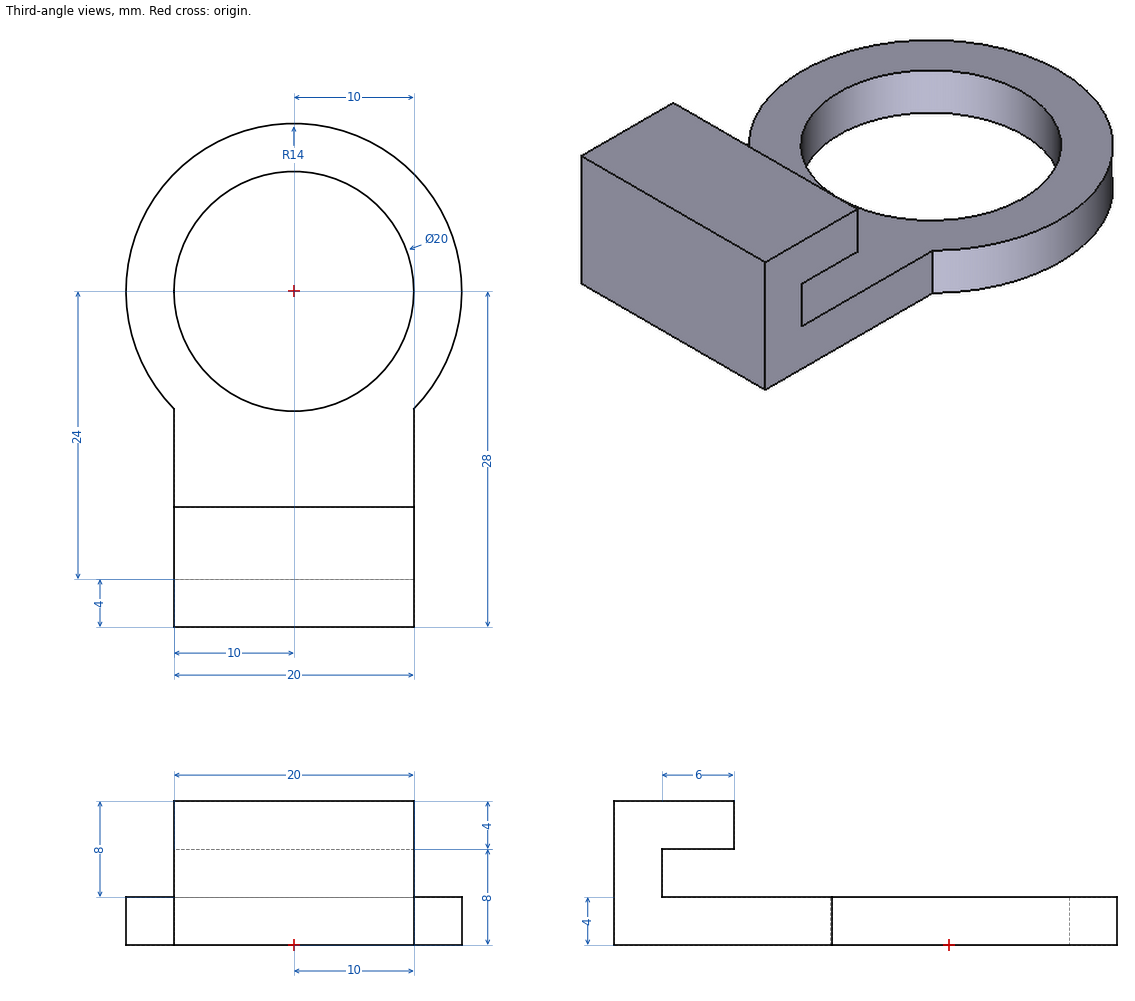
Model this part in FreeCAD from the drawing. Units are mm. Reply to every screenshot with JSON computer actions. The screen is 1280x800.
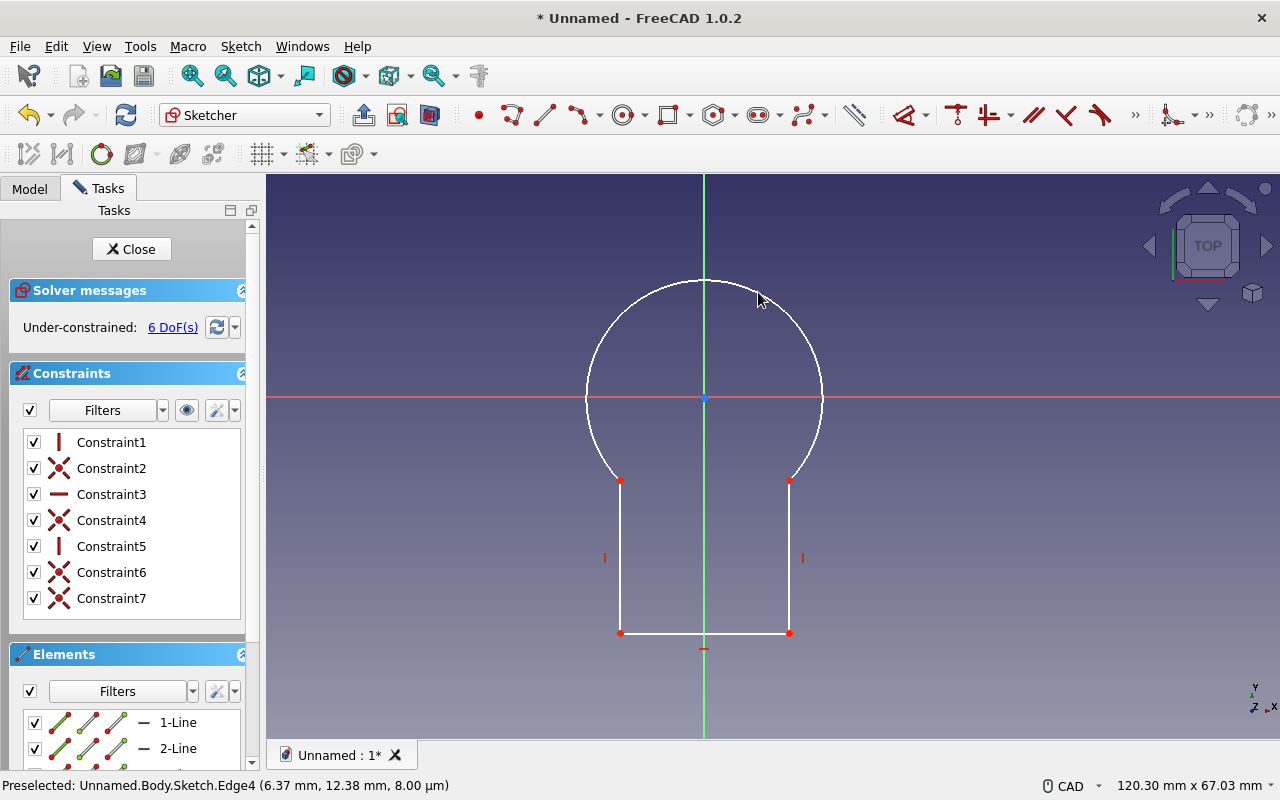
{"action": "left_click_drag", "start_coordinate": [694, 387], "coordinate": [714, 408]}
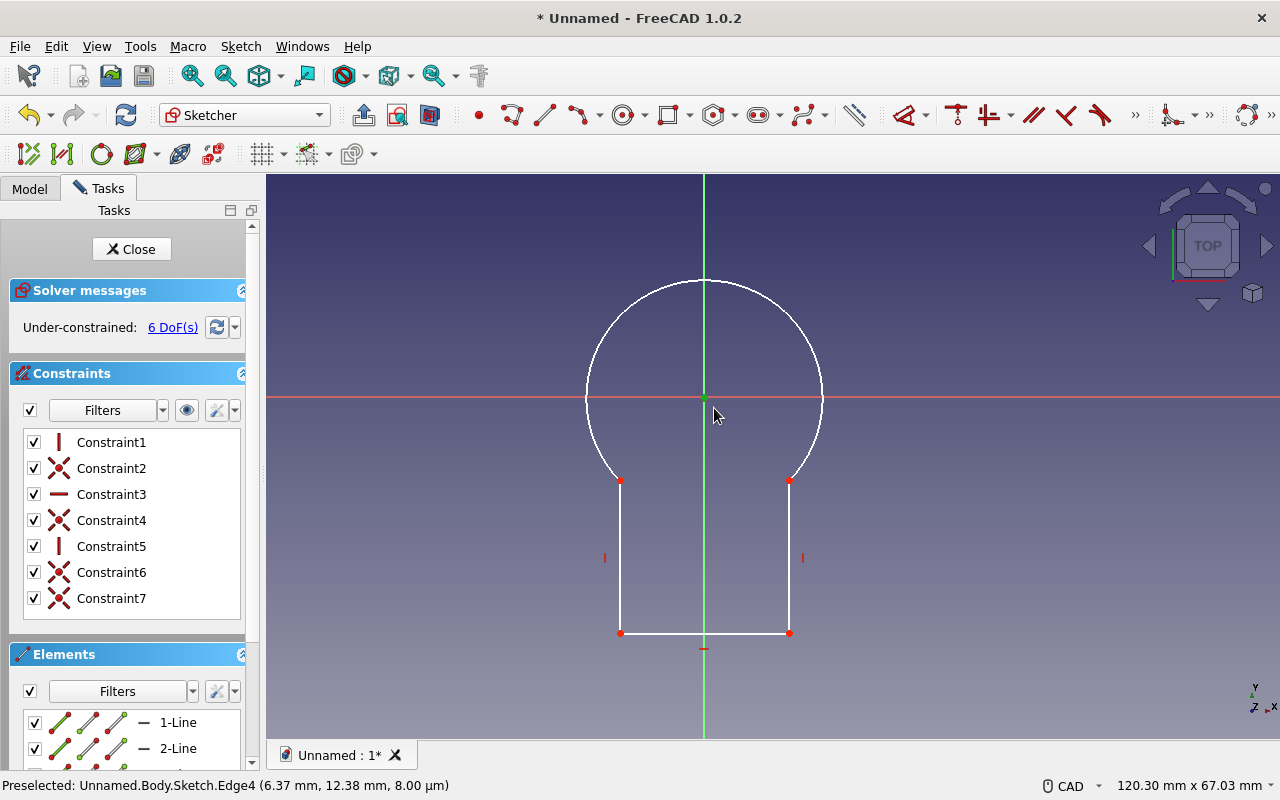
{"action": "left_click", "coordinate": [956, 116]}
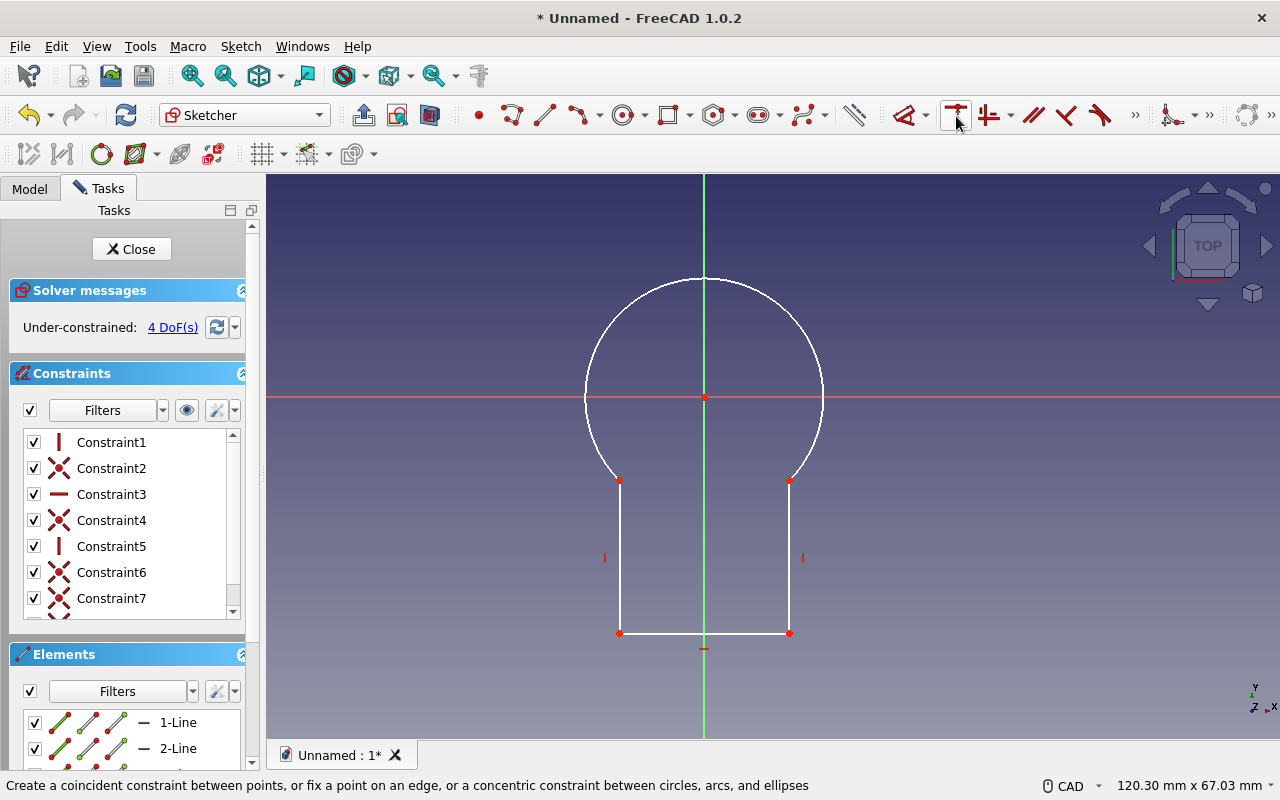
{"action": "left_click", "coordinate": [904, 116]}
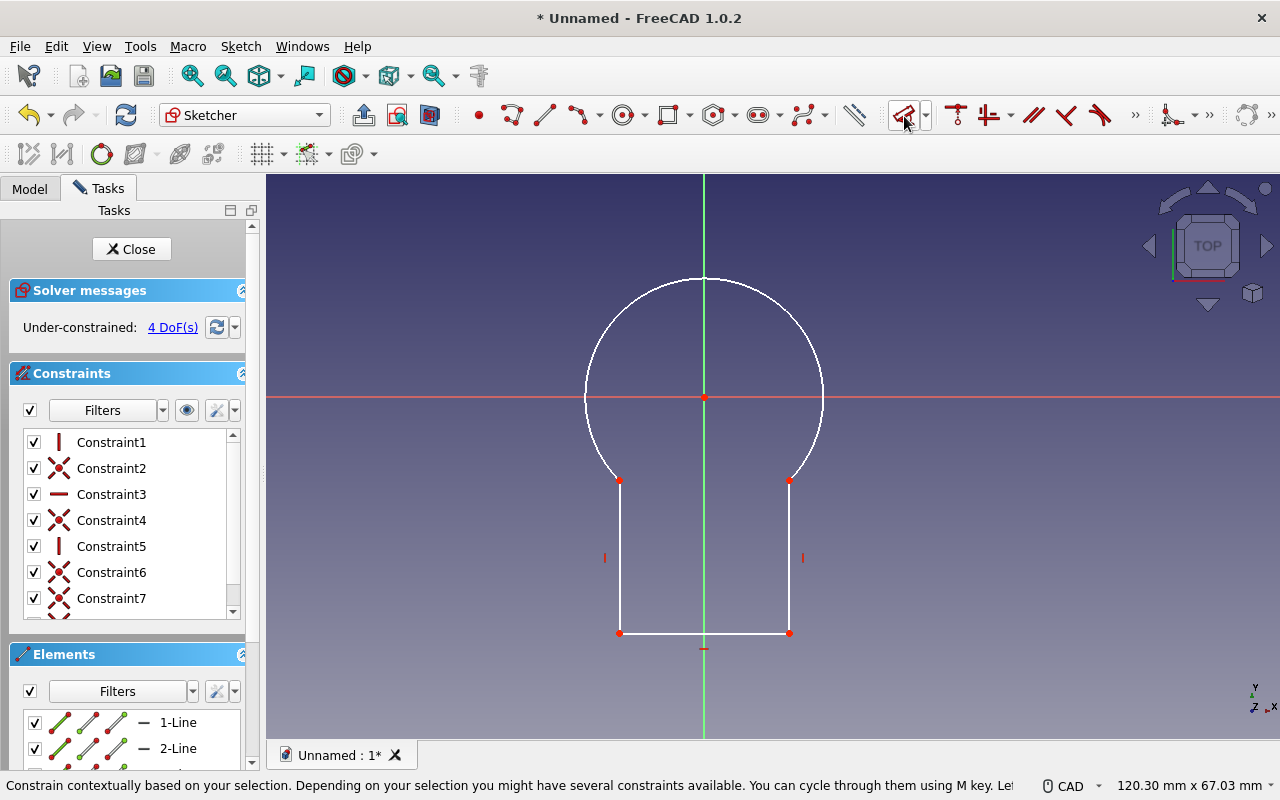
{"action": "left_click", "coordinate": [800, 327]}
{"action": "left_click", "coordinate": [826, 308]}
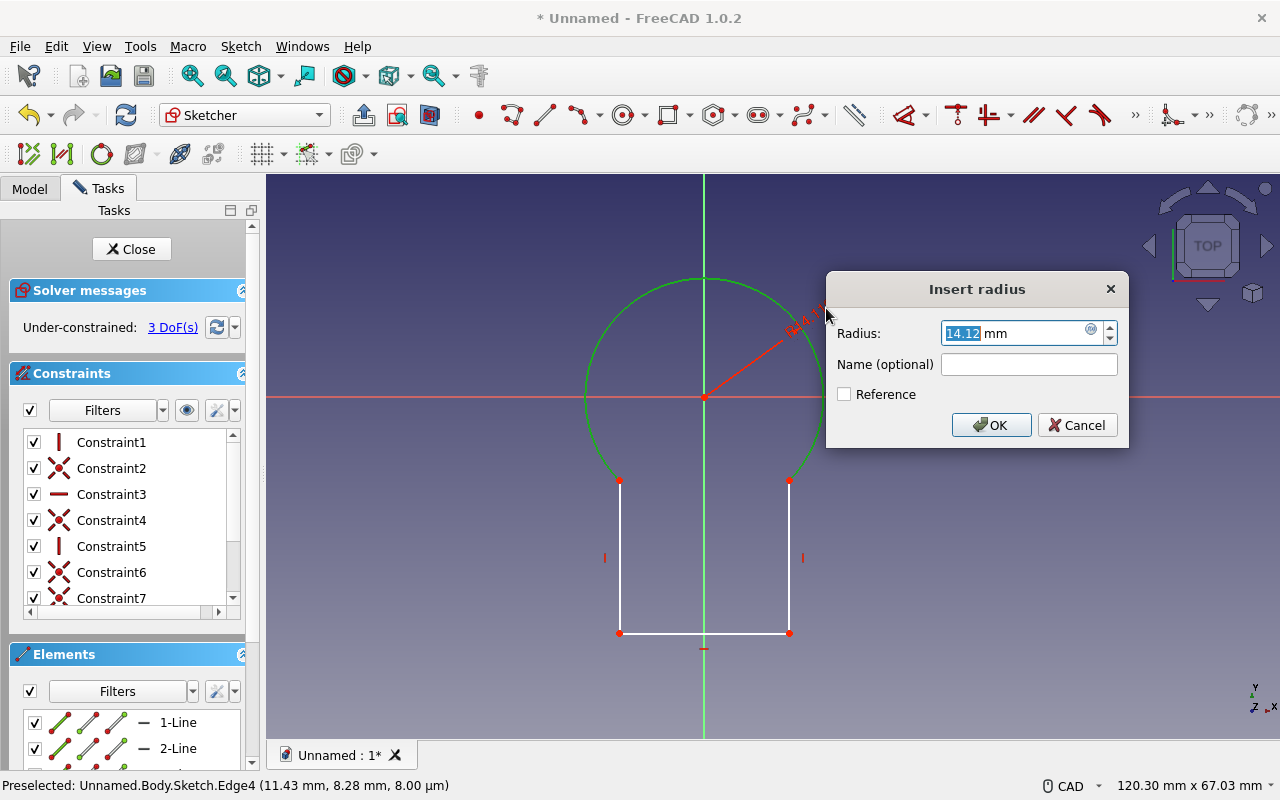
{"action": "type", "text": "14"}
{"action": "key", "text": "Return"}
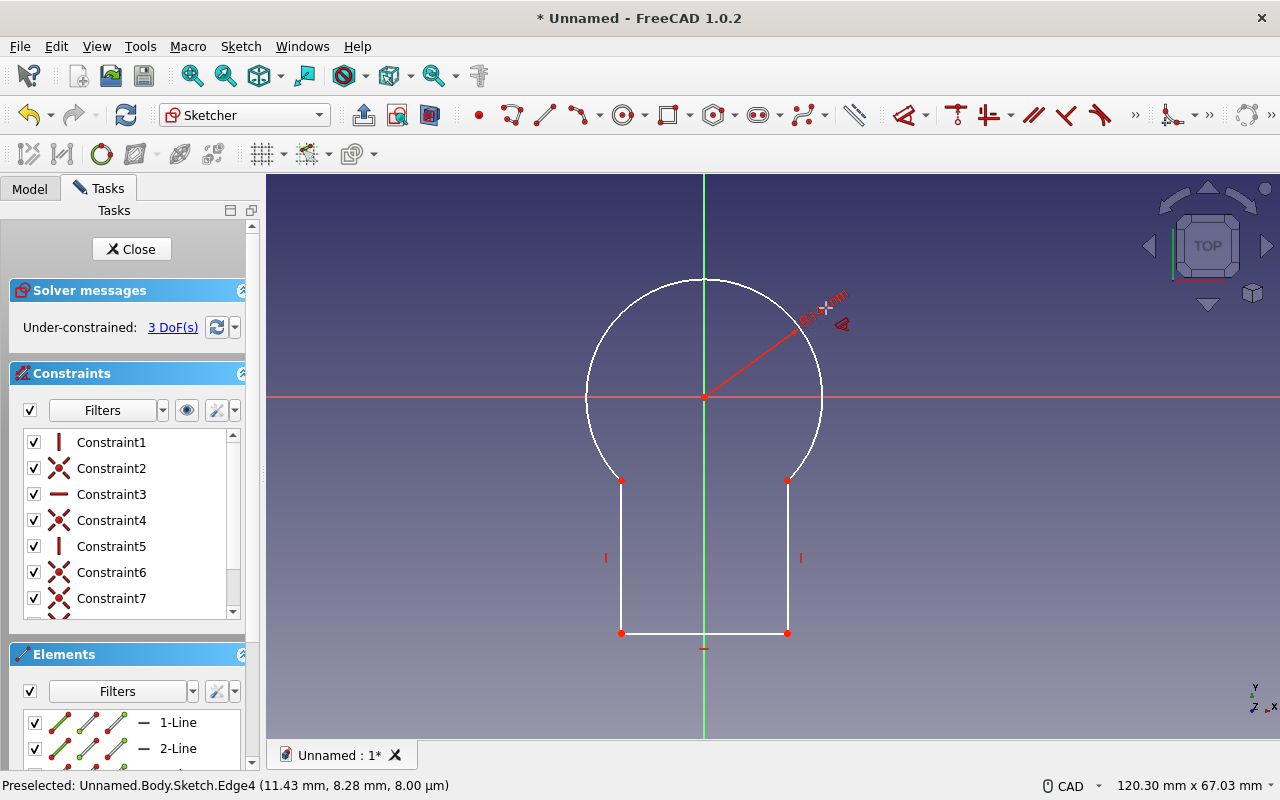
{"action": "left_click", "coordinate": [738, 634]}
{"action": "left_click", "coordinate": [666, 668]}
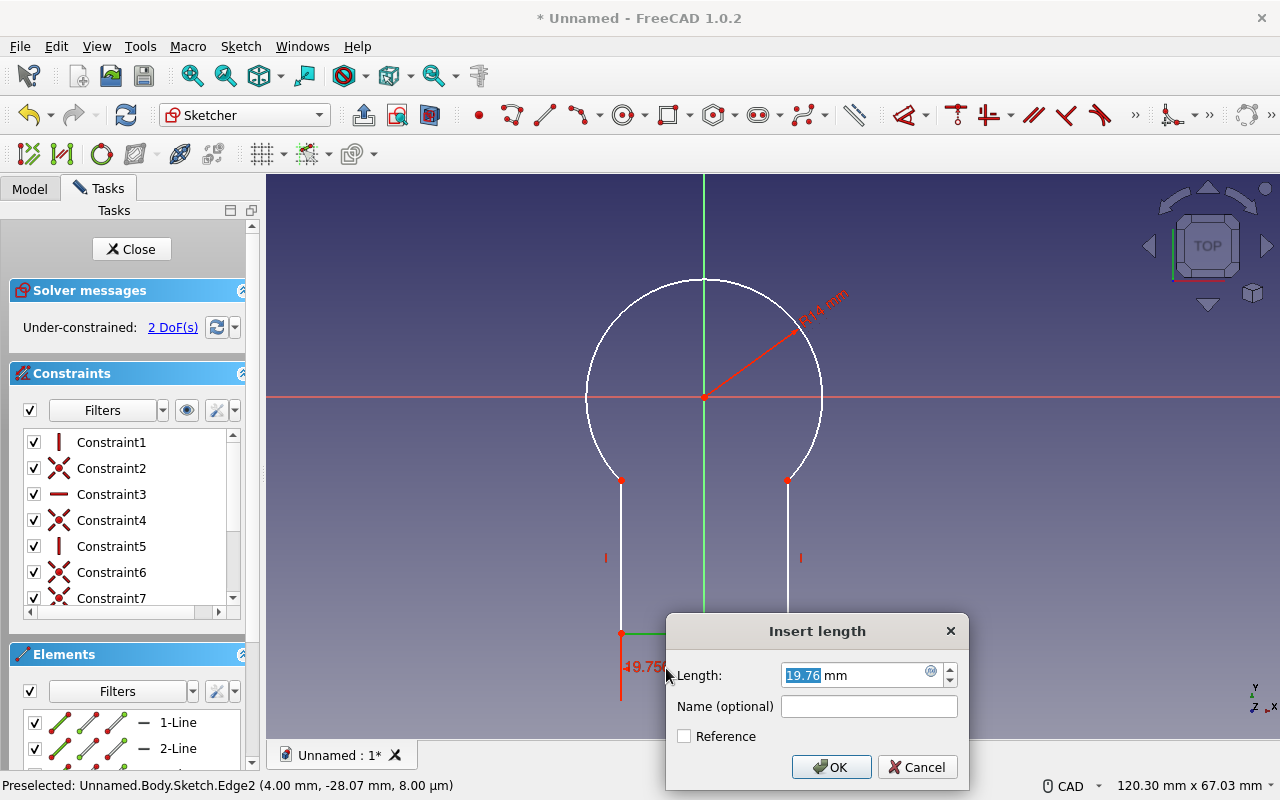
{"action": "type", "text": "20"}
{"action": "key", "text": "Return"}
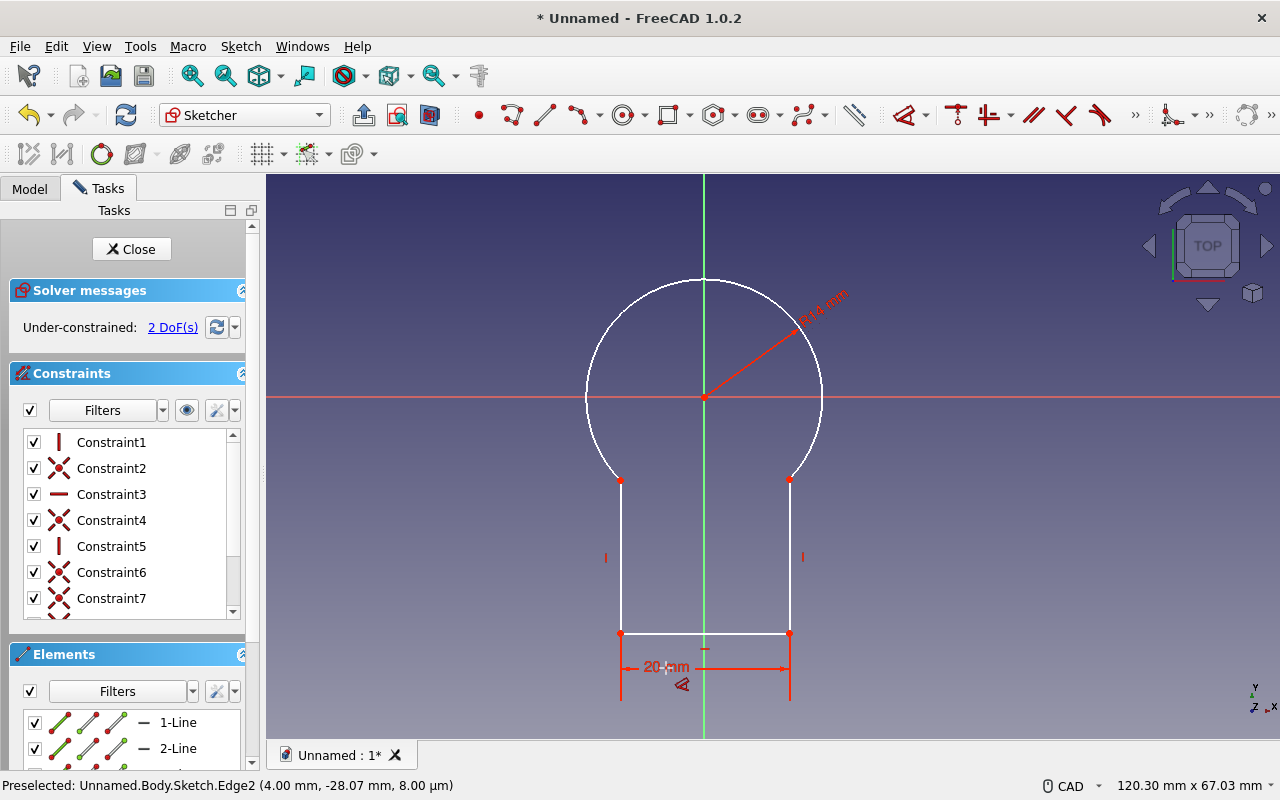
{"action": "left_click", "coordinate": [790, 479]}
{"action": "left_click", "coordinate": [747, 363]}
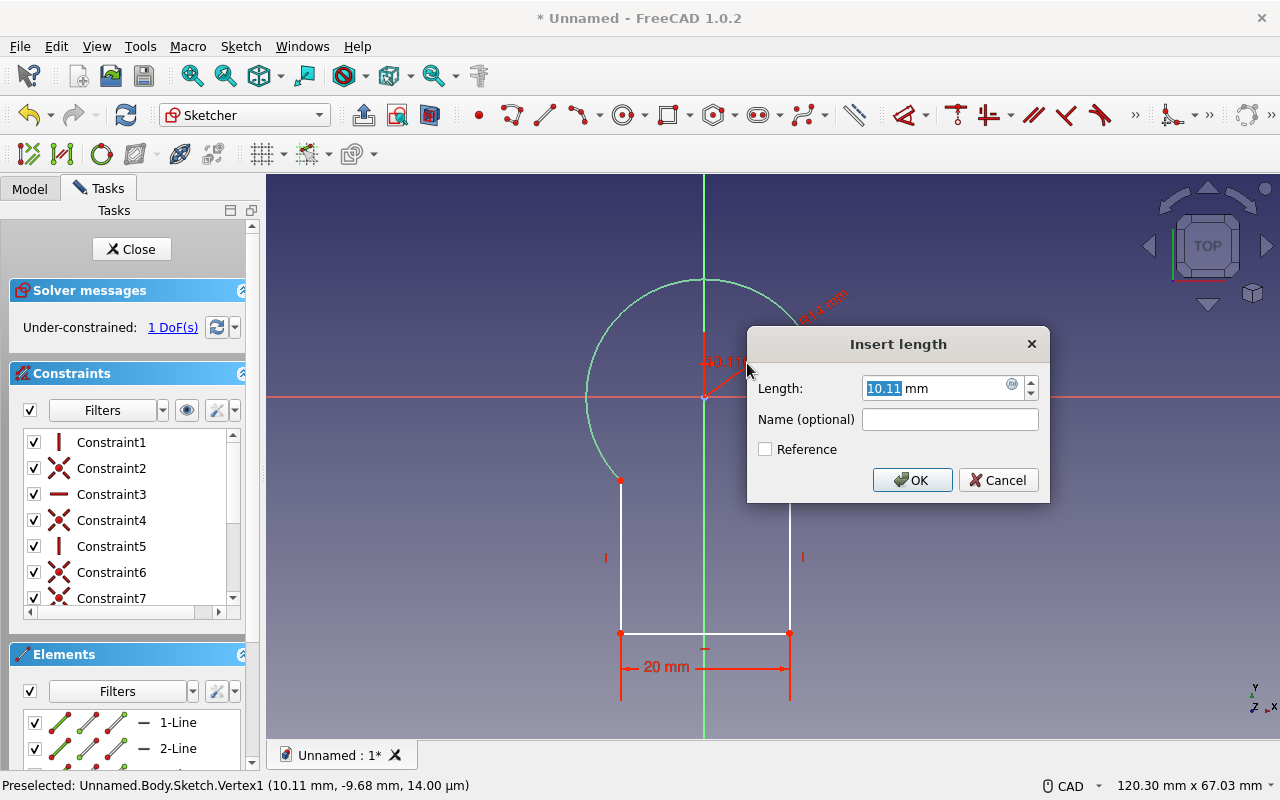
{"action": "type", "text": "10"}
{"action": "key", "text": "Return"}